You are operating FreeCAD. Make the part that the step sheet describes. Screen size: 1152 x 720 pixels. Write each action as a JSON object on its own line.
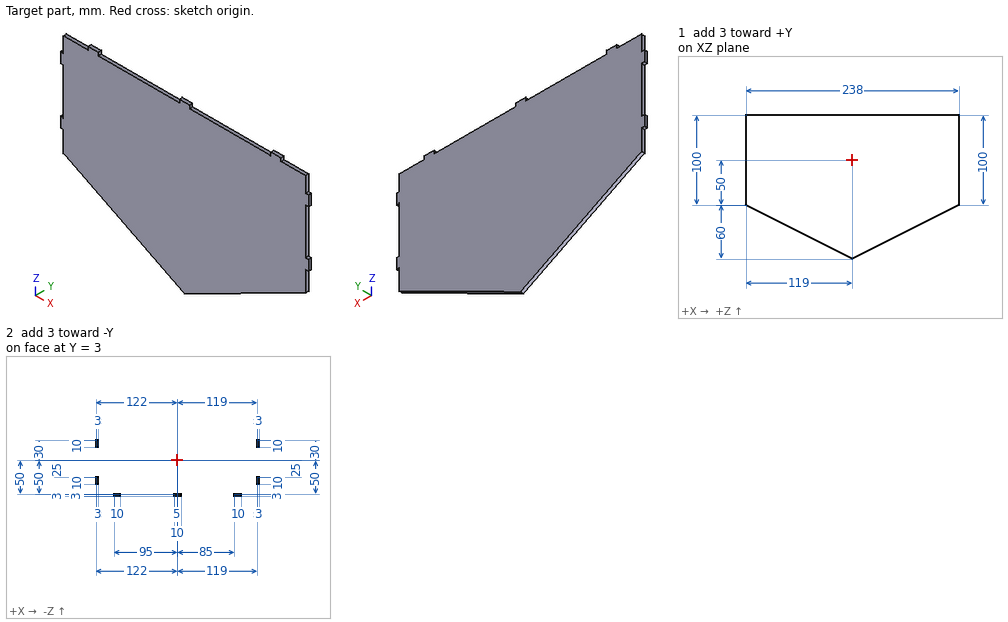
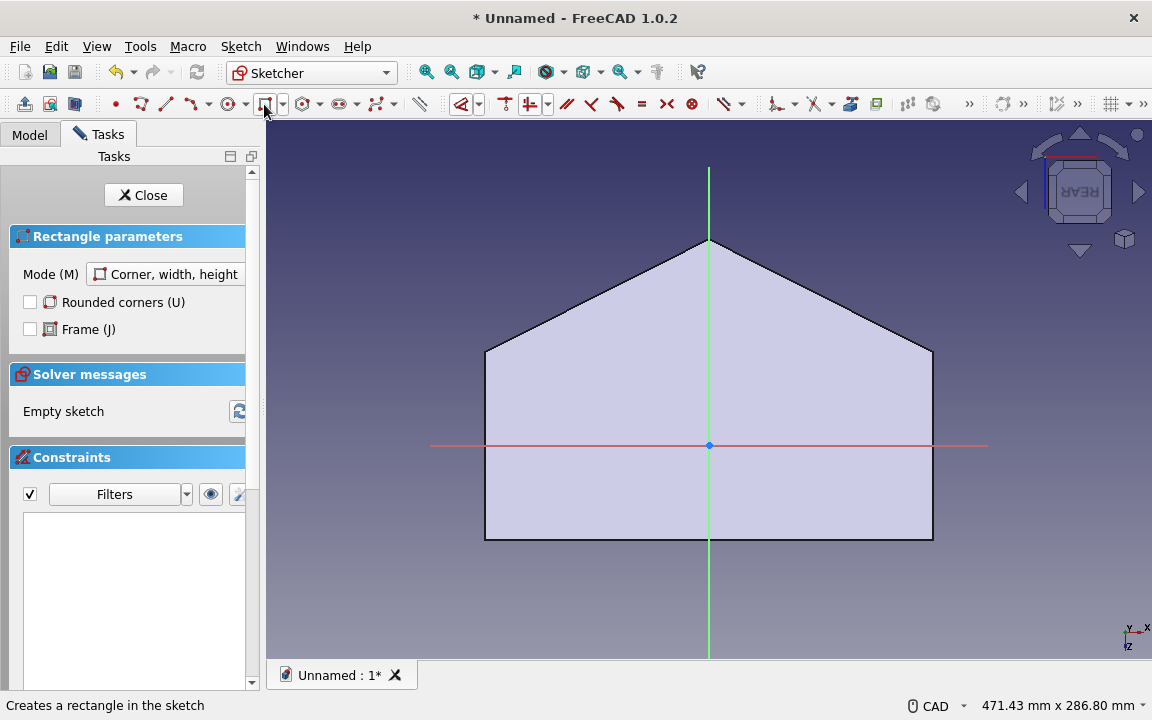
{"action": "scroll", "coordinate": [933, 390], "scroll_direction": "up", "scroll_amount": 6}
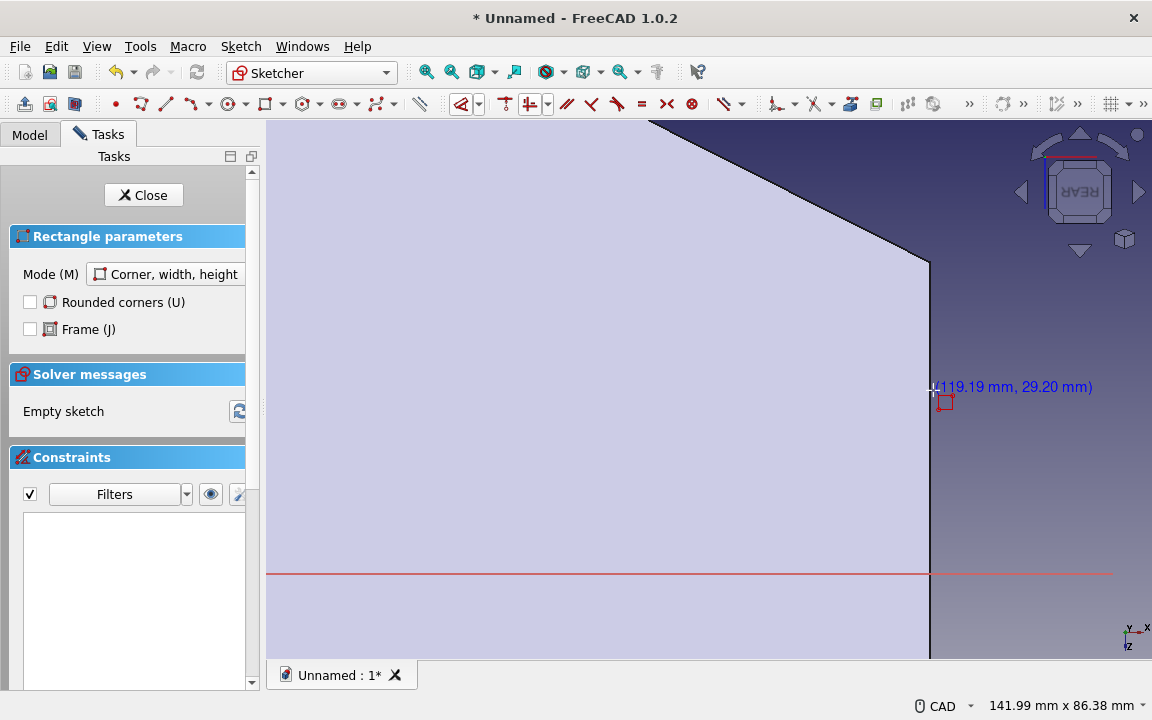
{"action": "left_click", "coordinate": [930, 387]}
{"action": "left_click", "coordinate": [949, 450]}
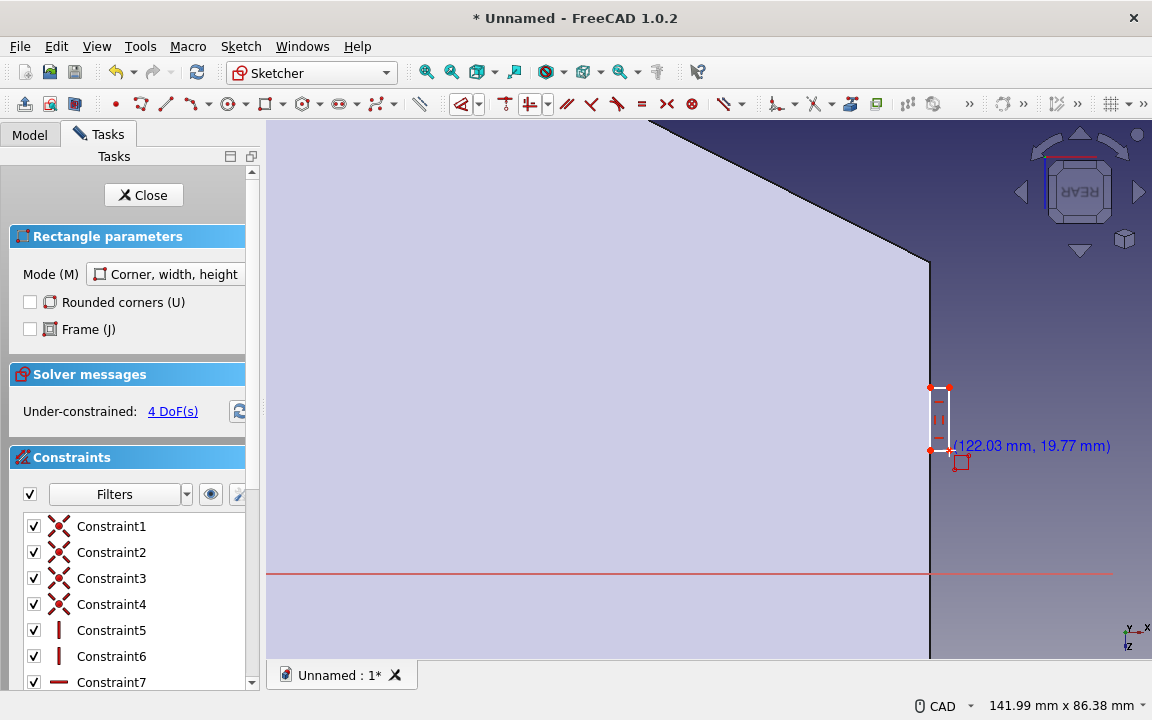
{"action": "scroll", "coordinate": [836, 279], "scroll_direction": "down", "scroll_amount": 6}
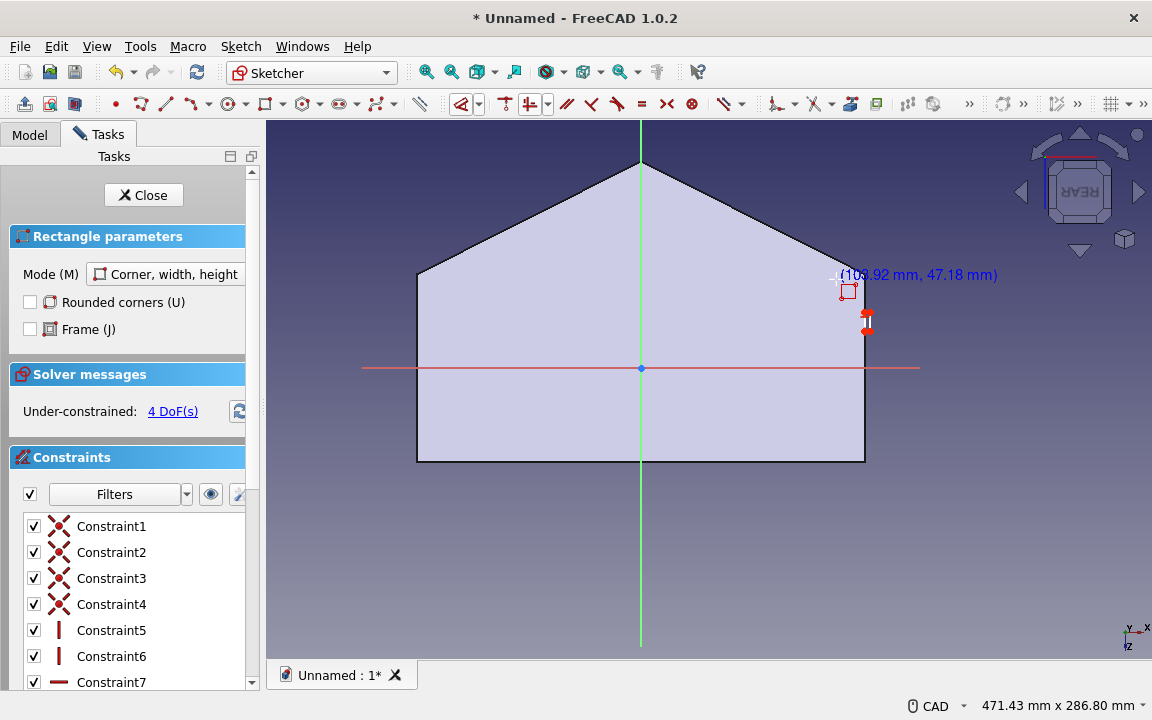
{"action": "scroll", "coordinate": [865, 415], "scroll_direction": "up", "scroll_amount": 6}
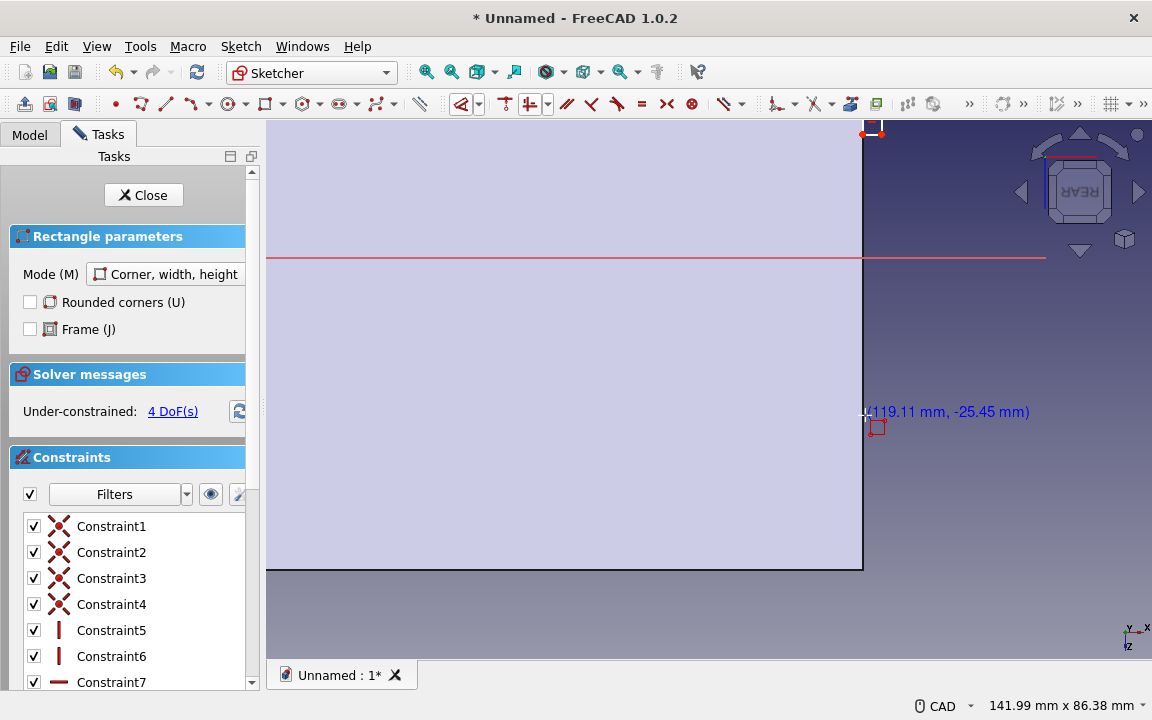
{"action": "left_click", "coordinate": [863, 414]}
{"action": "left_click", "coordinate": [881, 477]}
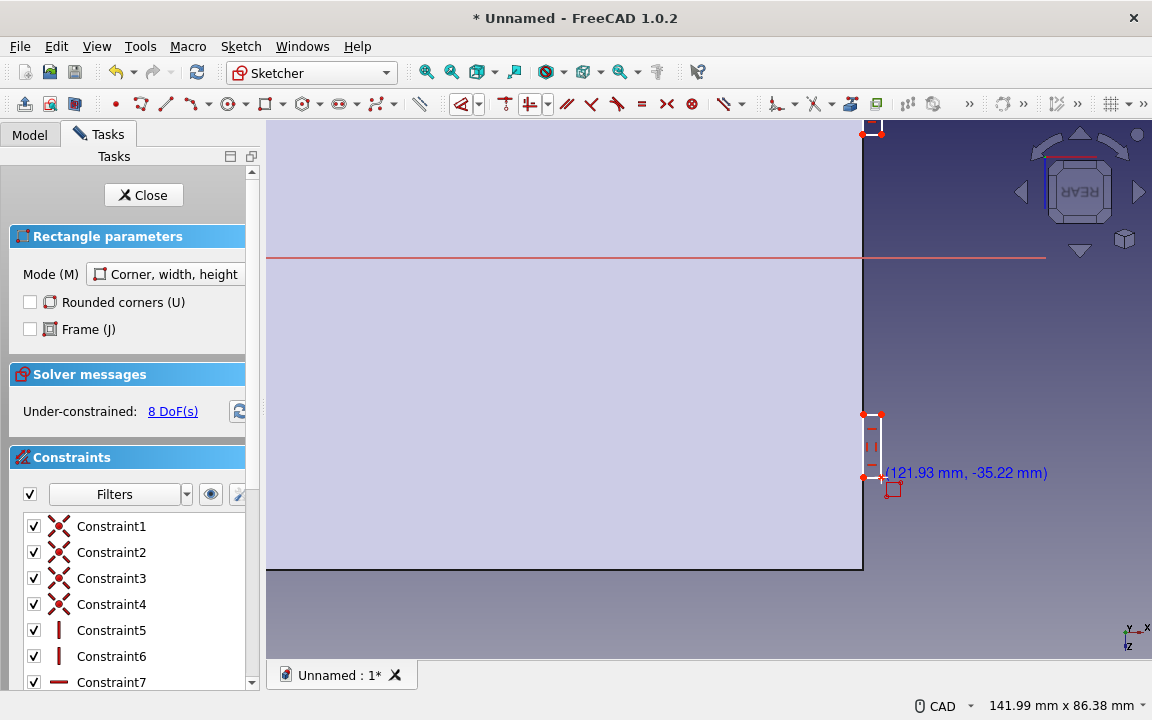
{"action": "scroll", "coordinate": [865, 415], "scroll_direction": "down", "scroll_amount": 6}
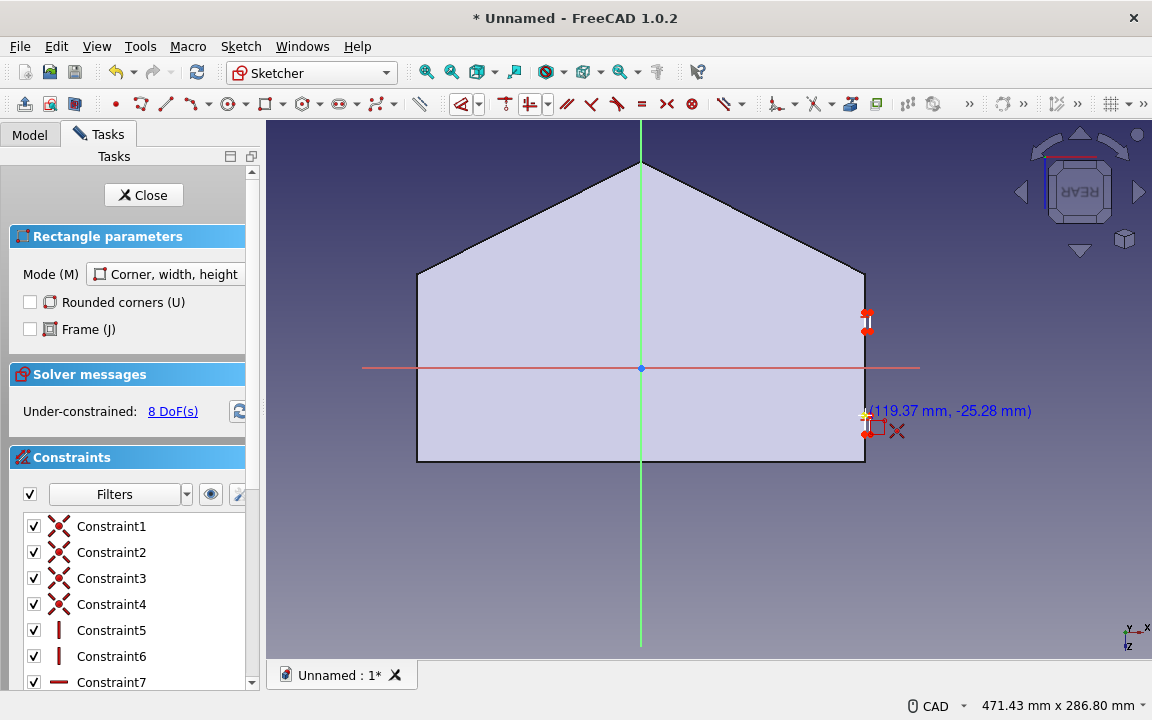
{"action": "scroll", "coordinate": [412, 415], "scroll_direction": "up", "scroll_amount": 6}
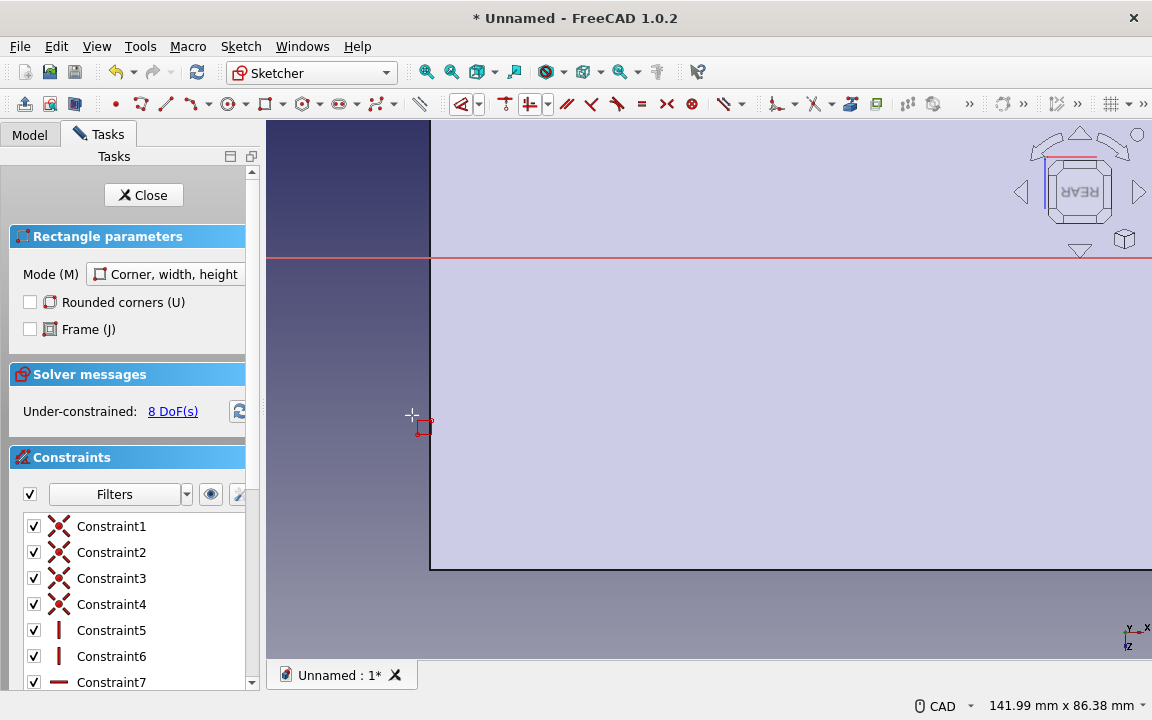
{"action": "left_click", "coordinate": [411, 414]}
{"action": "left_click", "coordinate": [430, 477]}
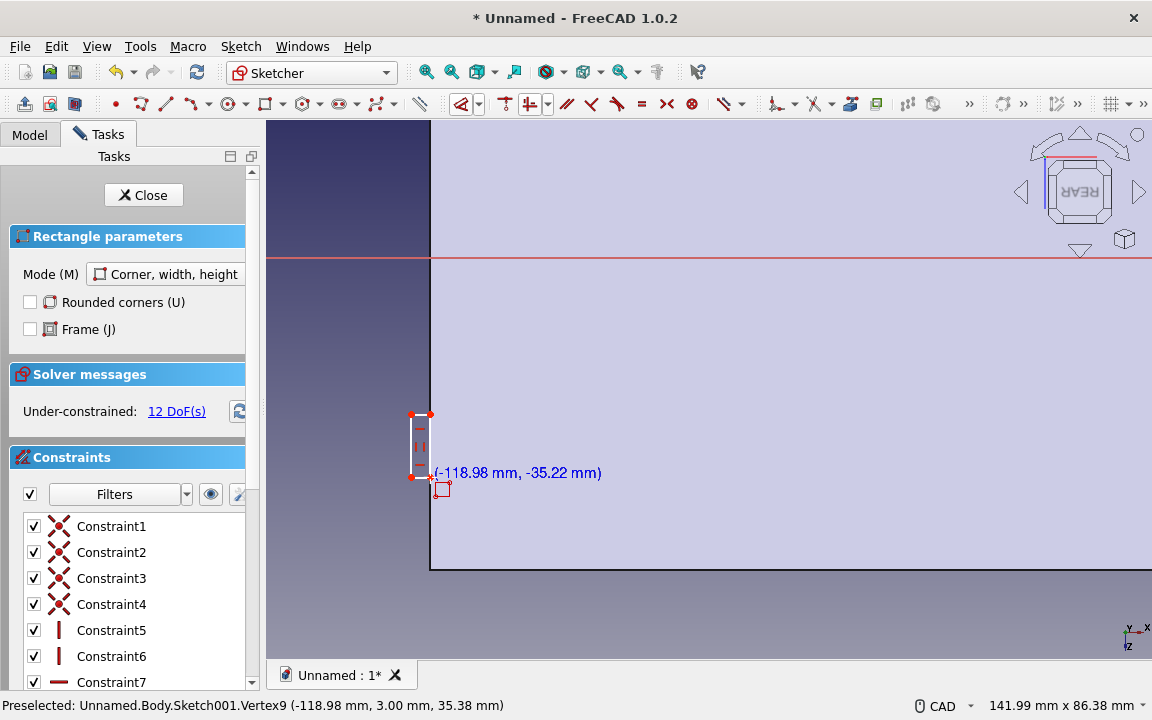
{"action": "scroll", "coordinate": [411, 415], "scroll_direction": "down", "scroll_amount": 6}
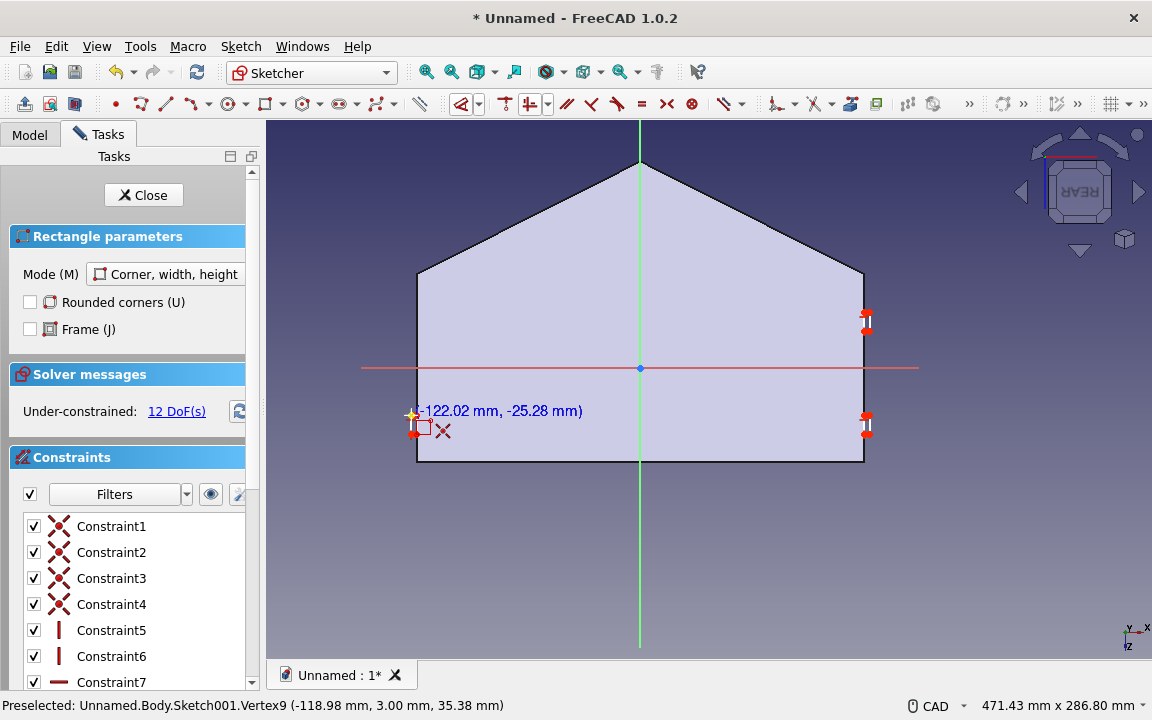
{"action": "scroll", "coordinate": [411, 312], "scroll_direction": "up", "scroll_amount": 6}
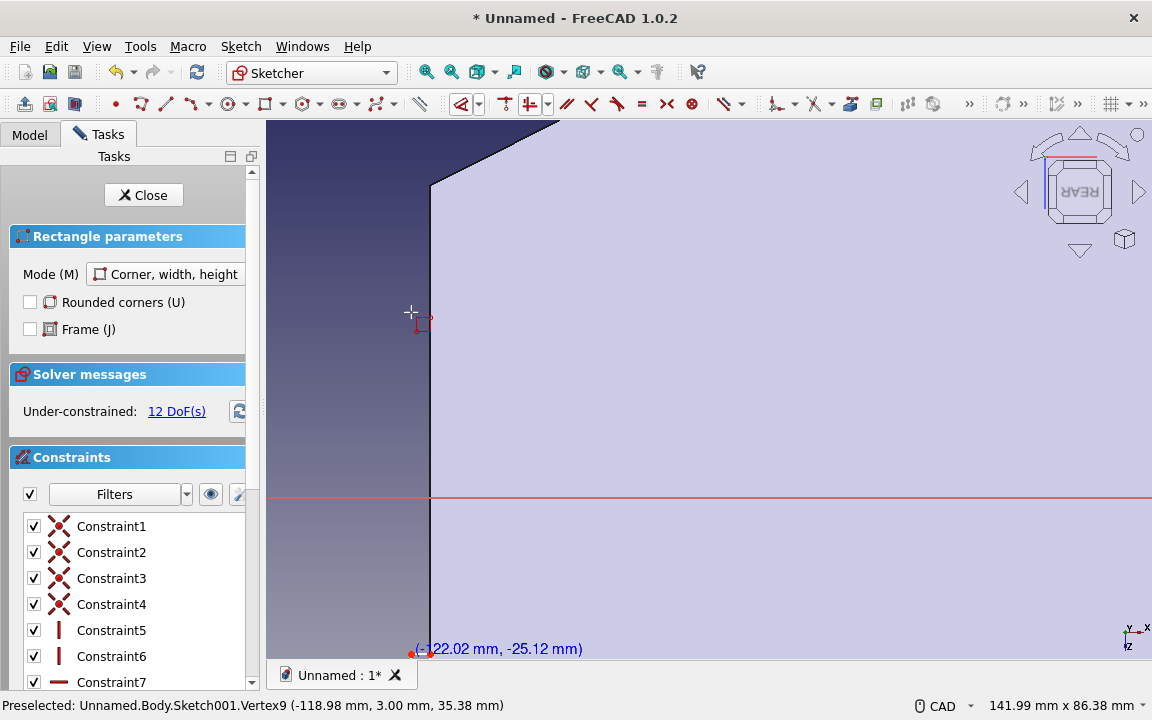
{"action": "left_click", "coordinate": [411, 310]}
{"action": "left_click", "coordinate": [430, 373]}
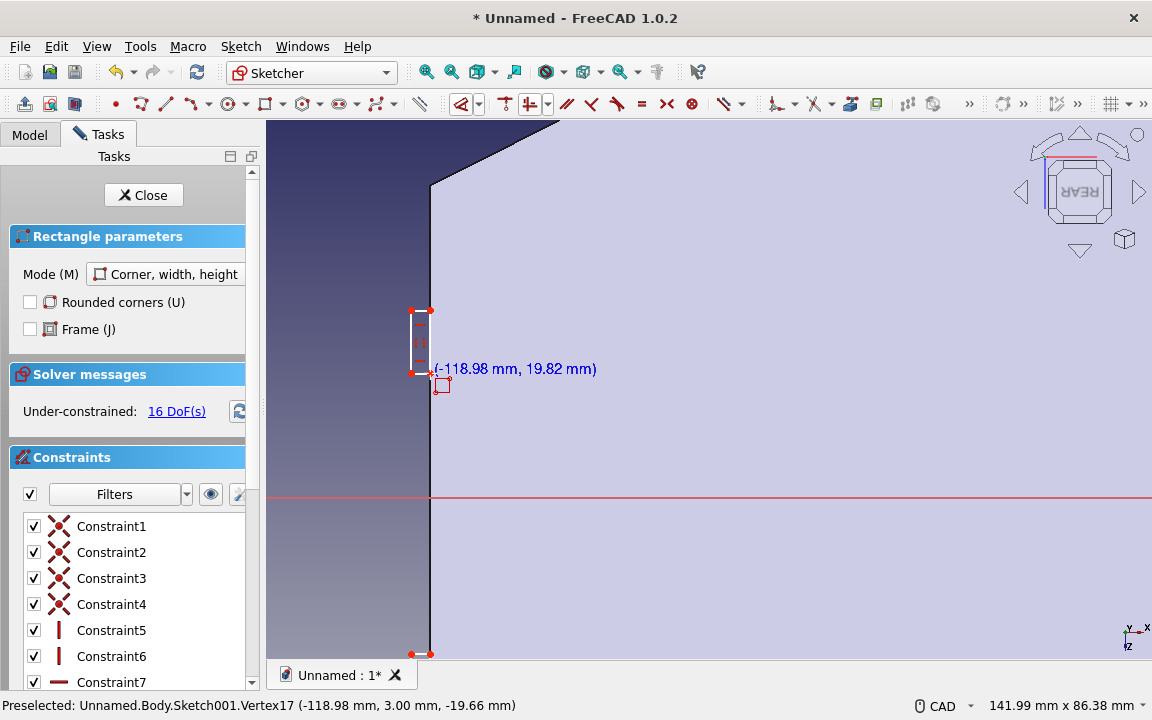
{"action": "scroll", "coordinate": [411, 312], "scroll_direction": "down", "scroll_amount": 6}